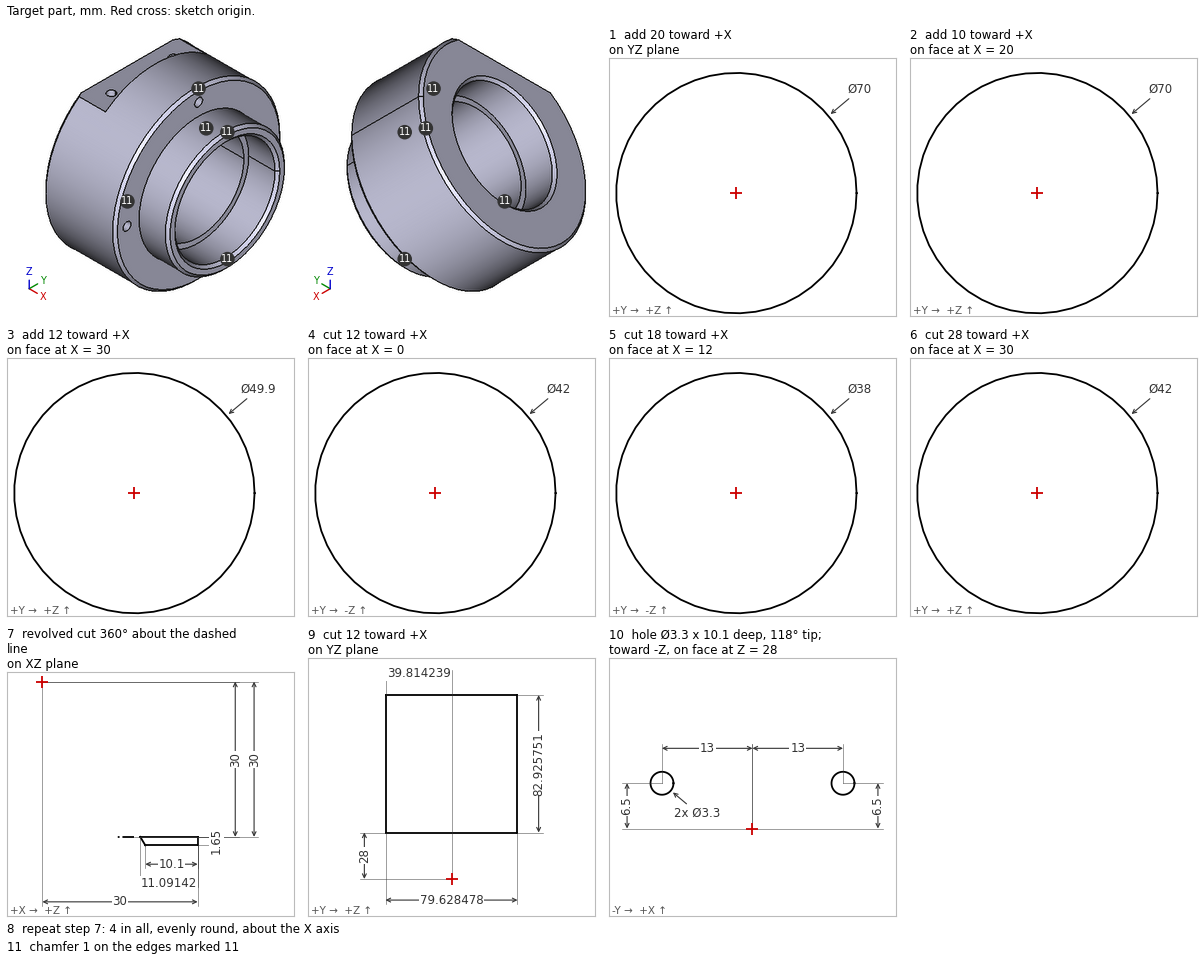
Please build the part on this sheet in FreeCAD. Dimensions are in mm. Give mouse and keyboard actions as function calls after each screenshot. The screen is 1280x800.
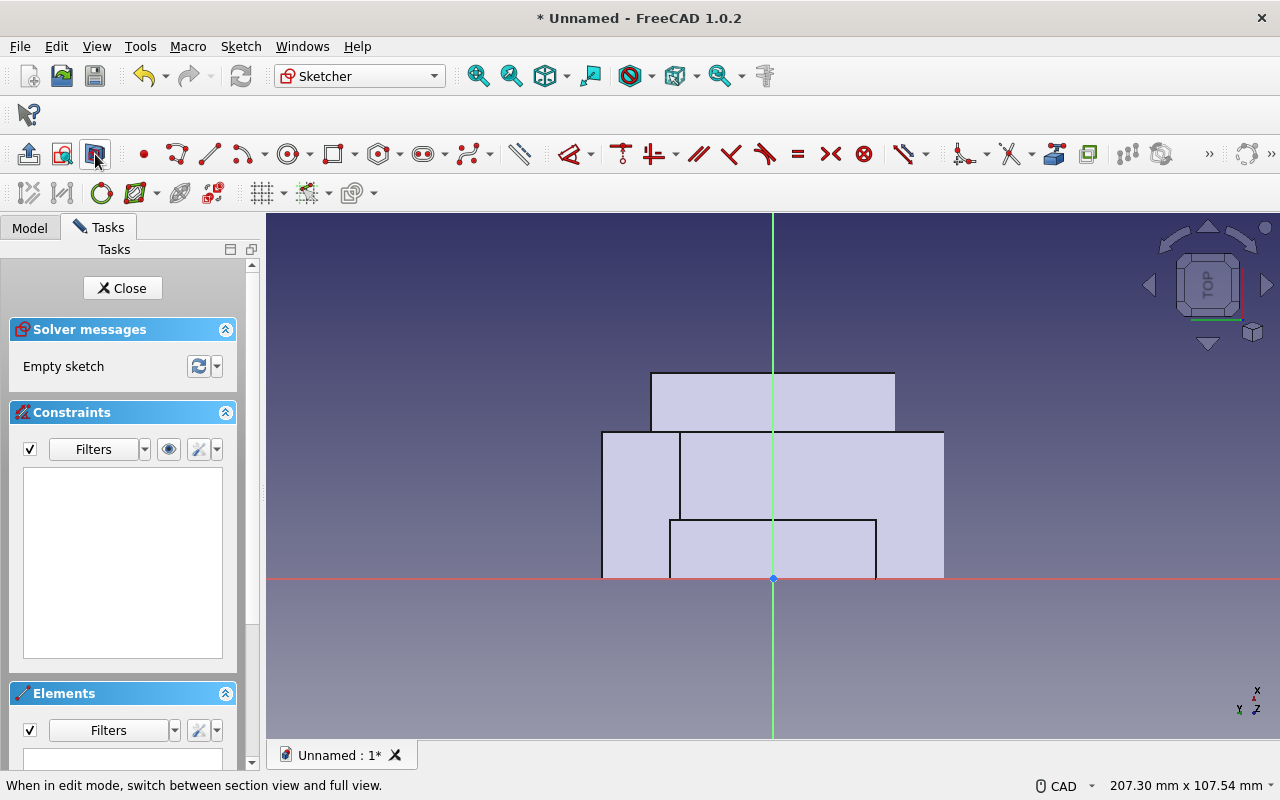
scroll(795, 586, up, 7)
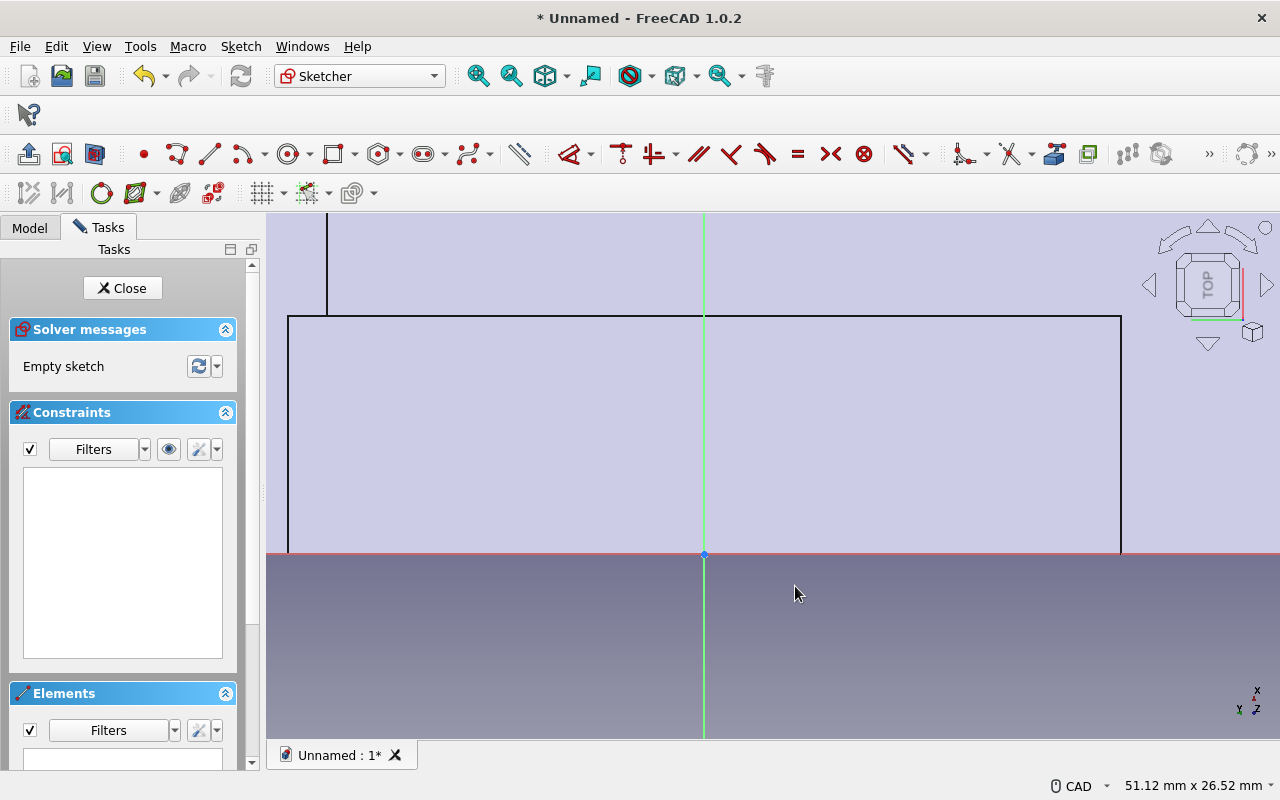
click(288, 154)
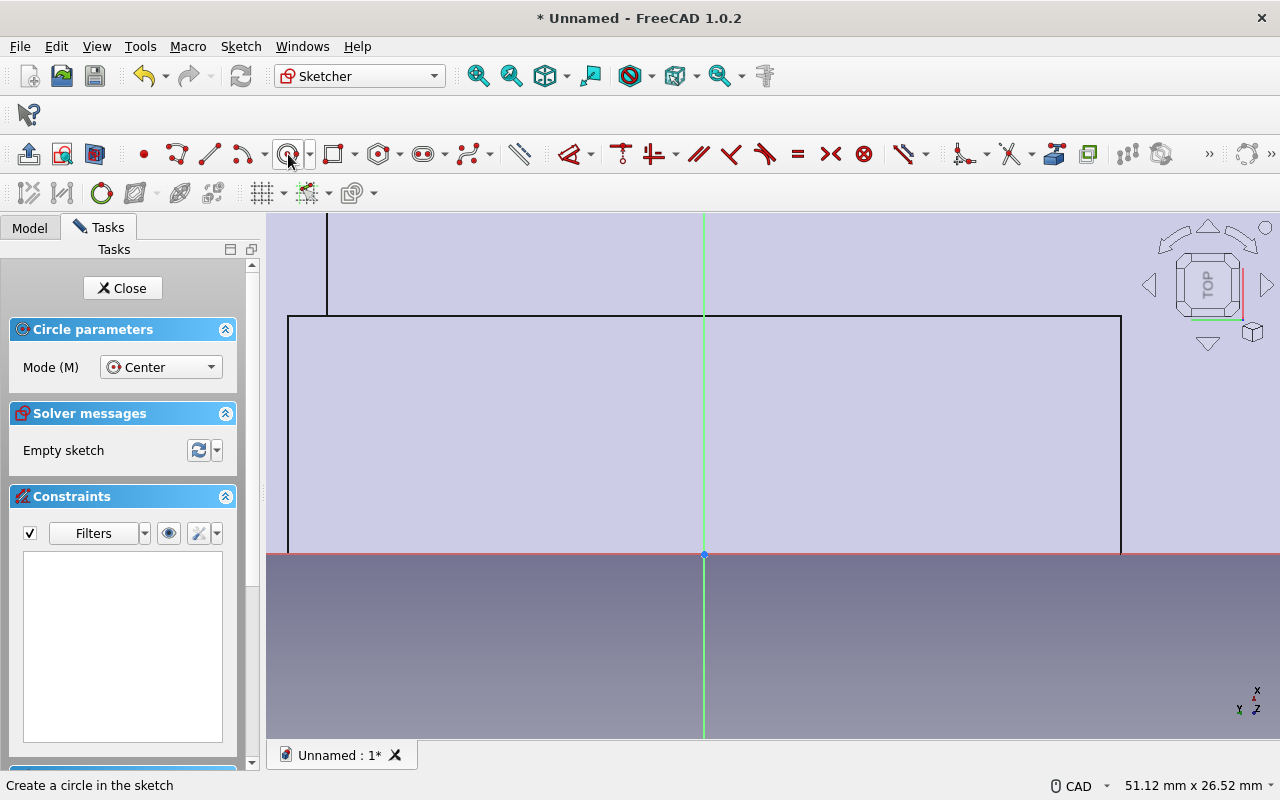
click(446, 425)
move(469, 402)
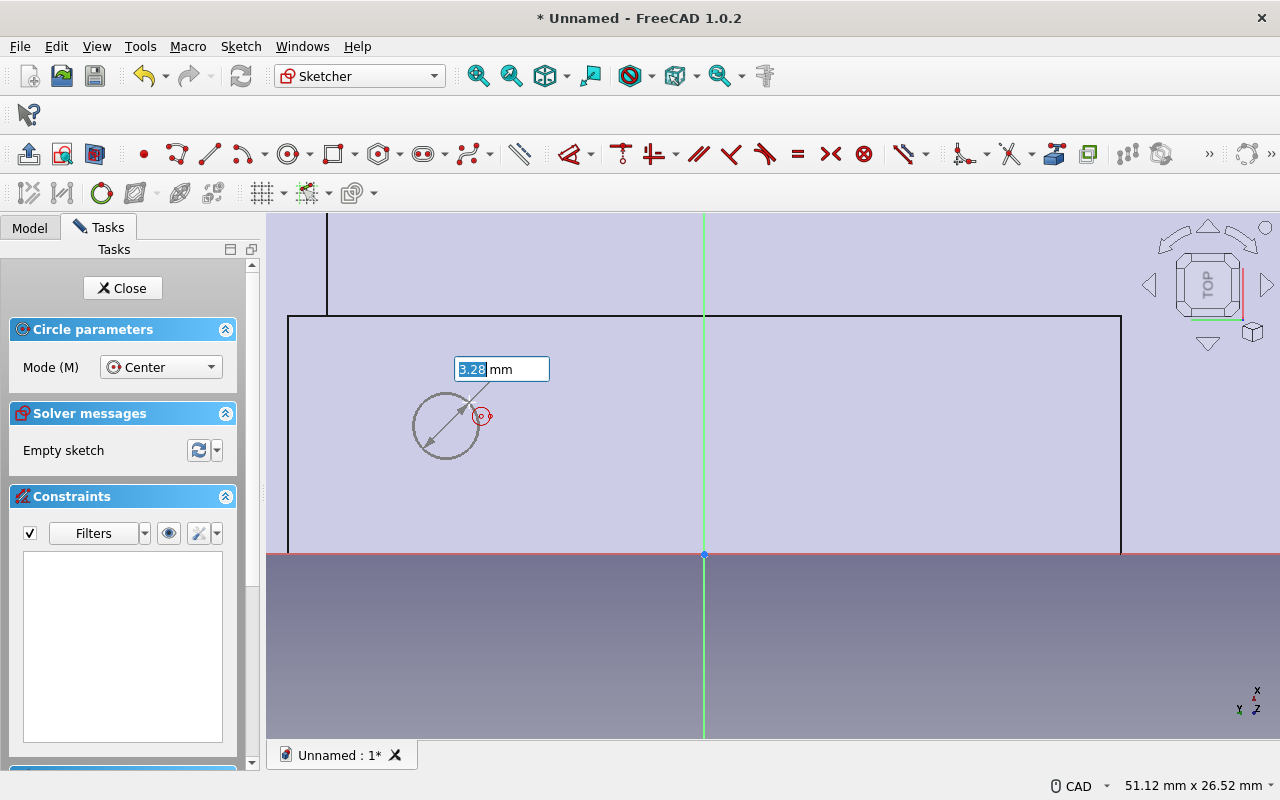
text(3.3)
key(Return)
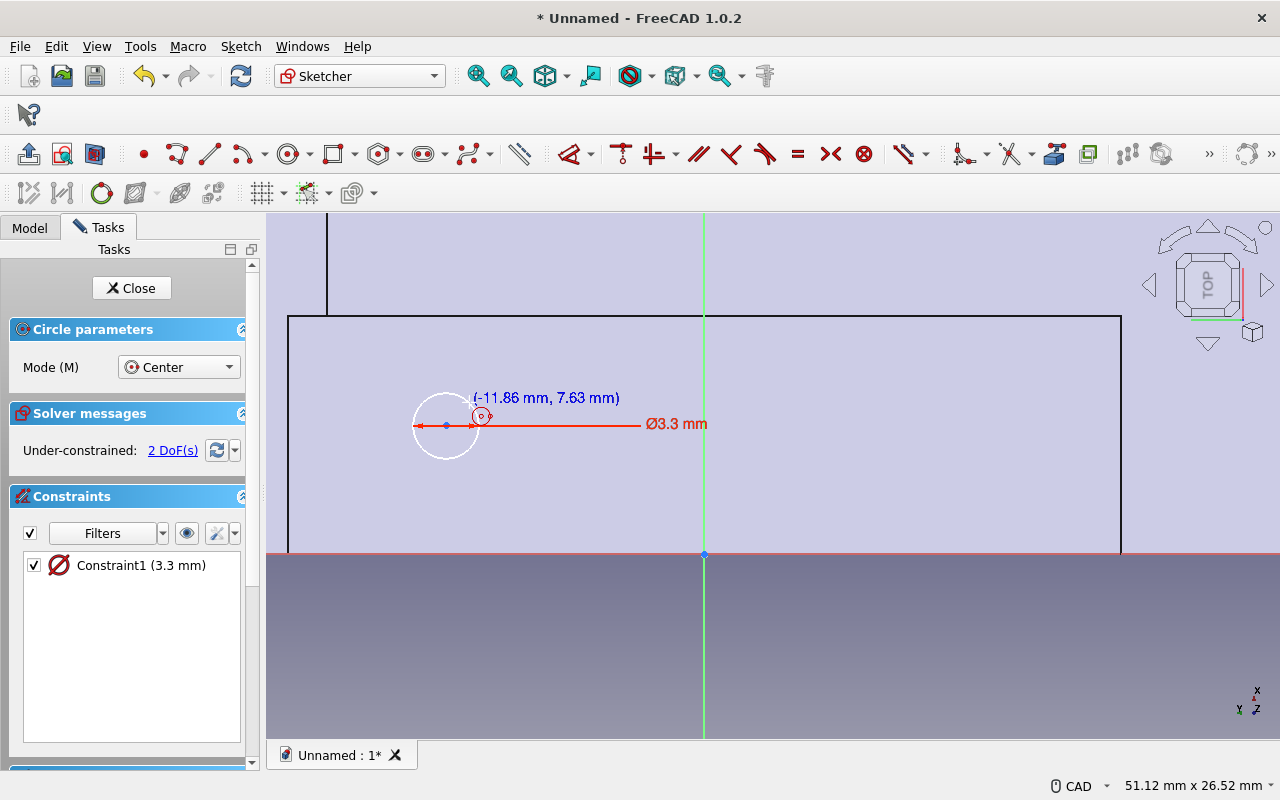
click(962, 425)
move(985, 402)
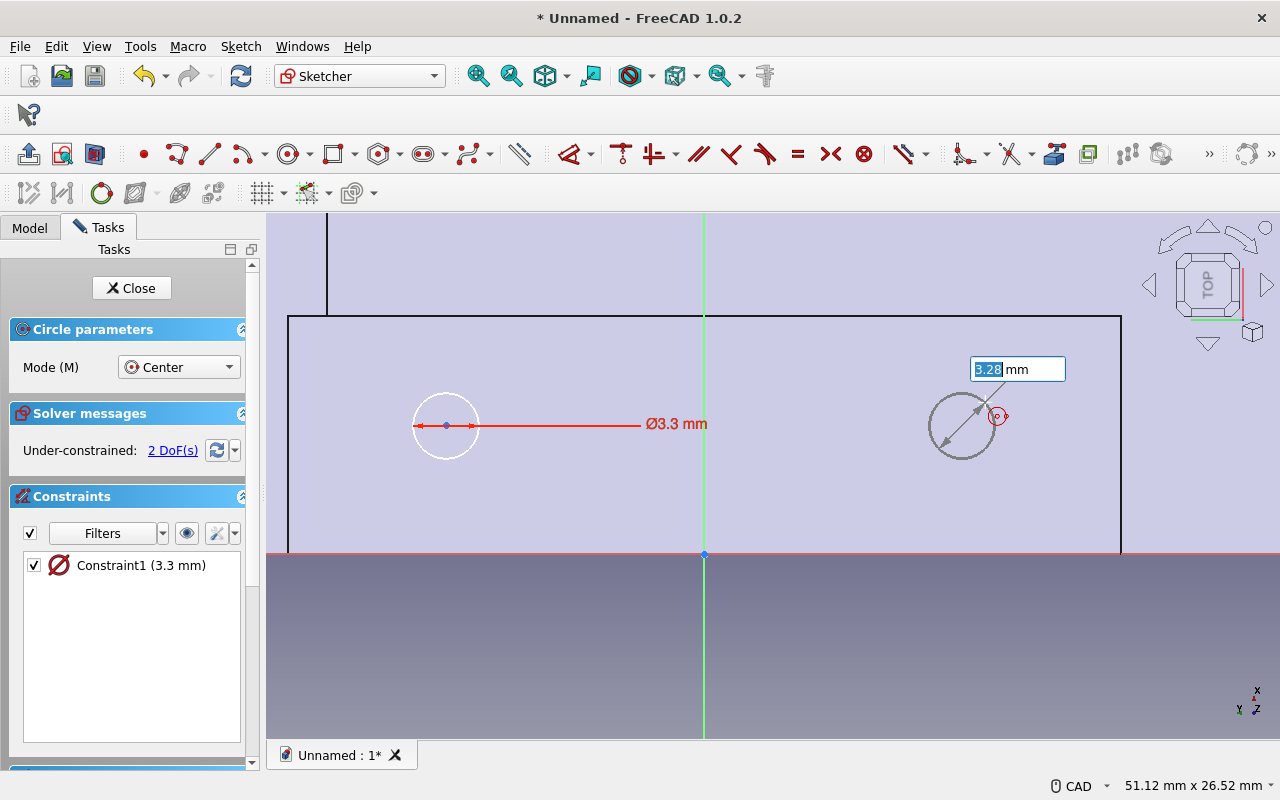
text(3.3)
key(Return)
key(Escape)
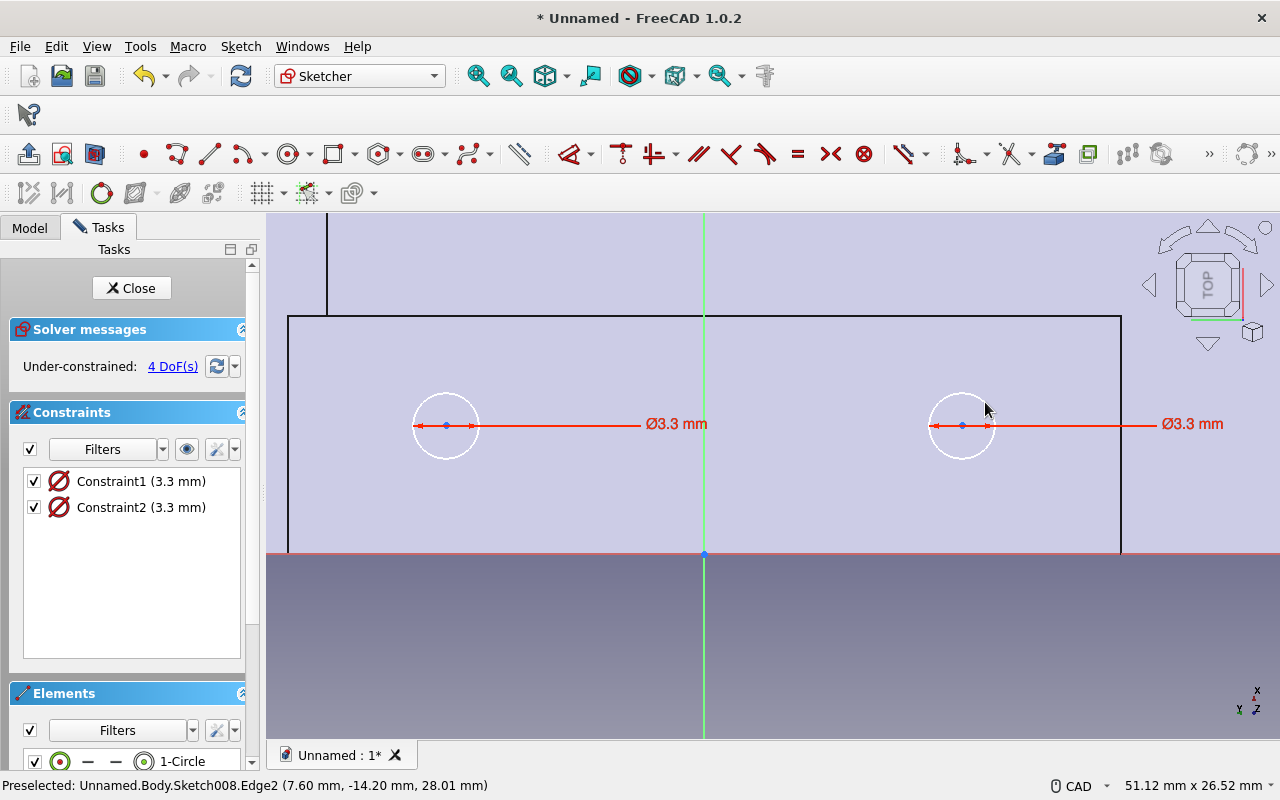
click(568, 154)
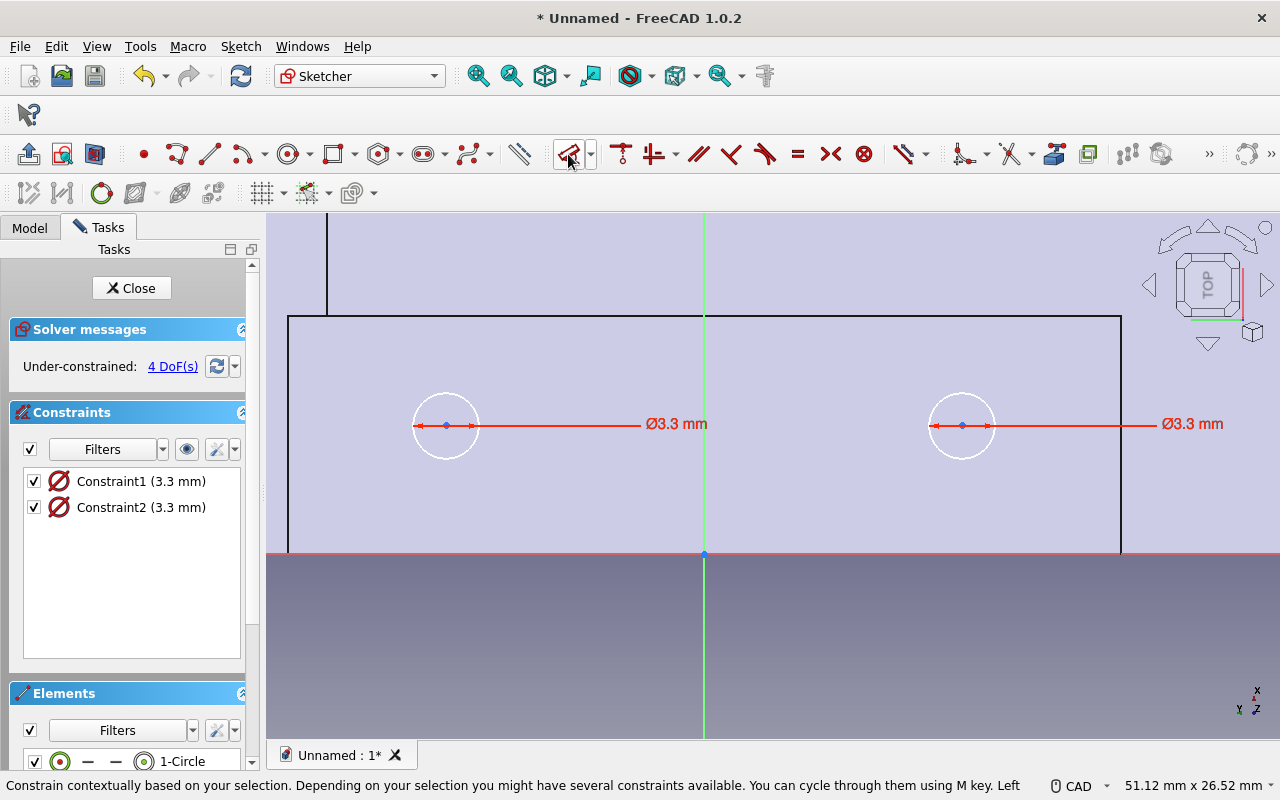
click(446, 426)
click(575, 588)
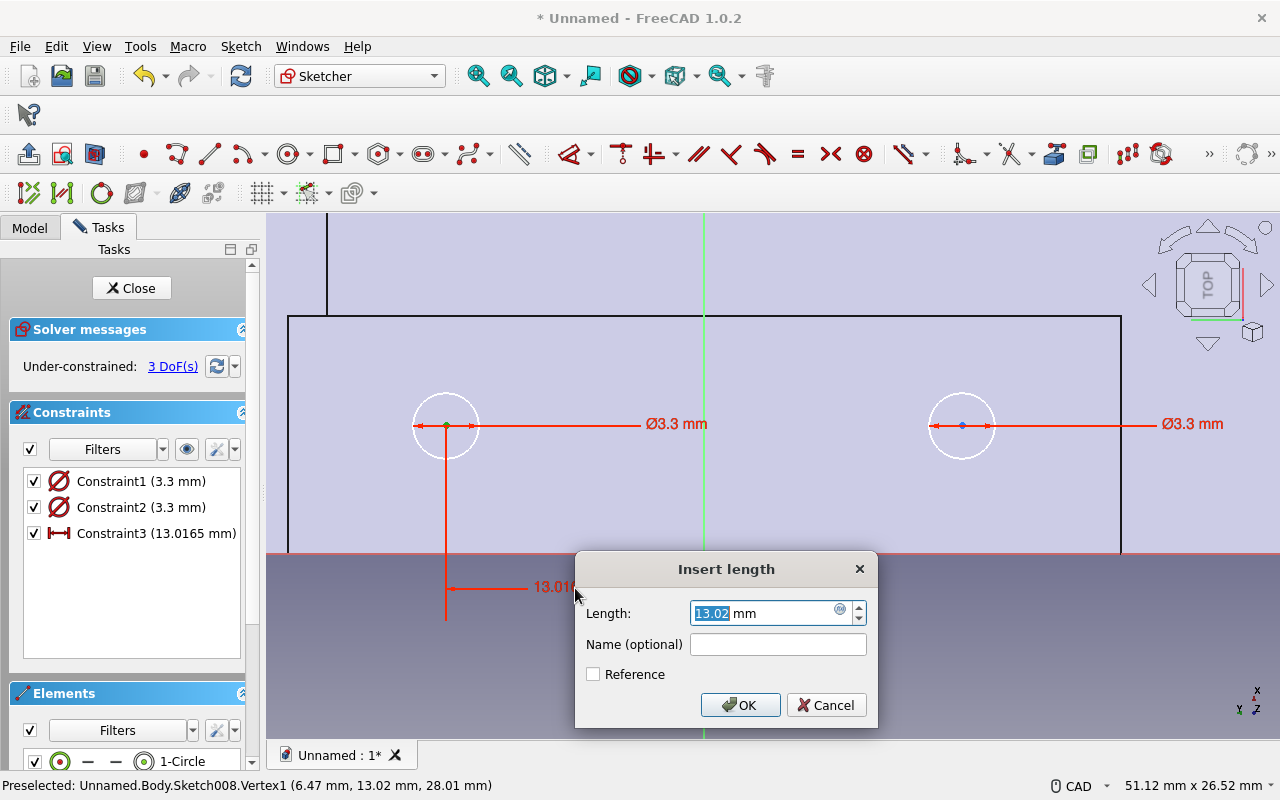
text(13)
key(Return)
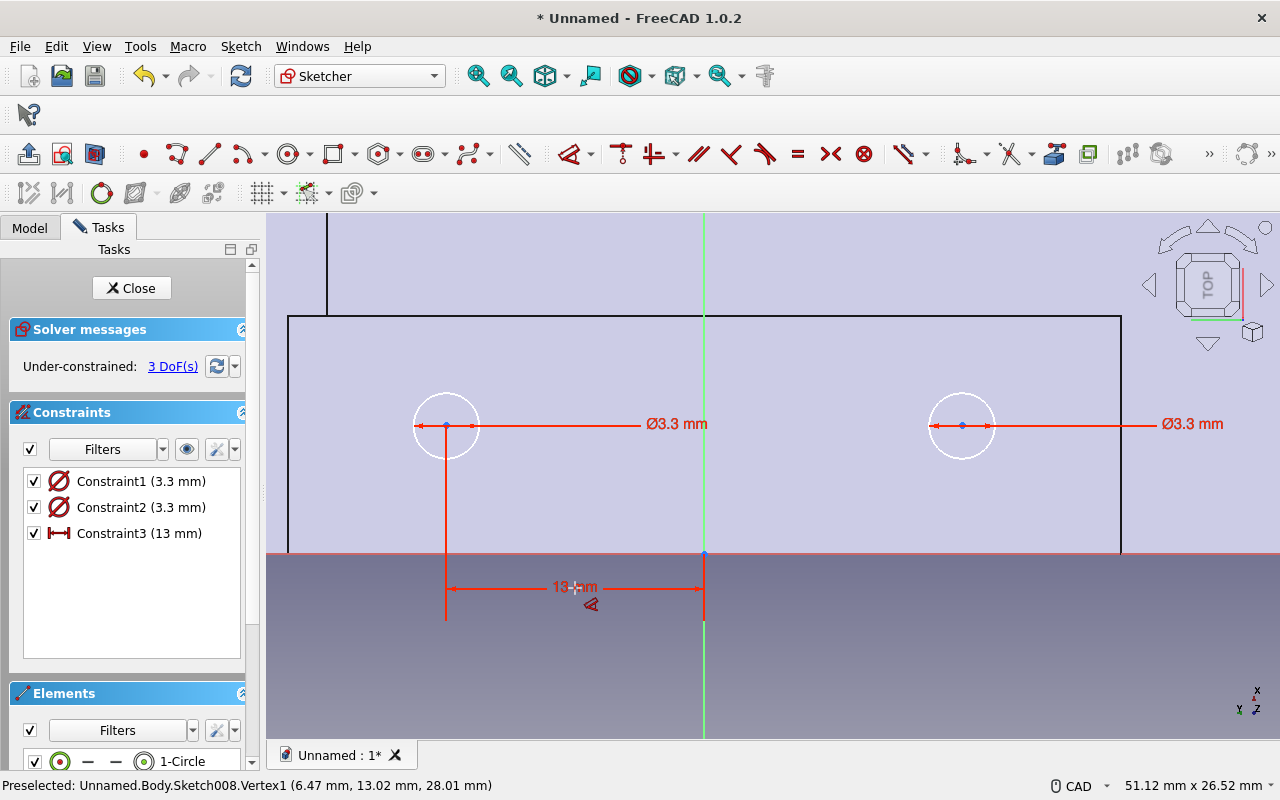
click(962, 426)
click(833, 588)